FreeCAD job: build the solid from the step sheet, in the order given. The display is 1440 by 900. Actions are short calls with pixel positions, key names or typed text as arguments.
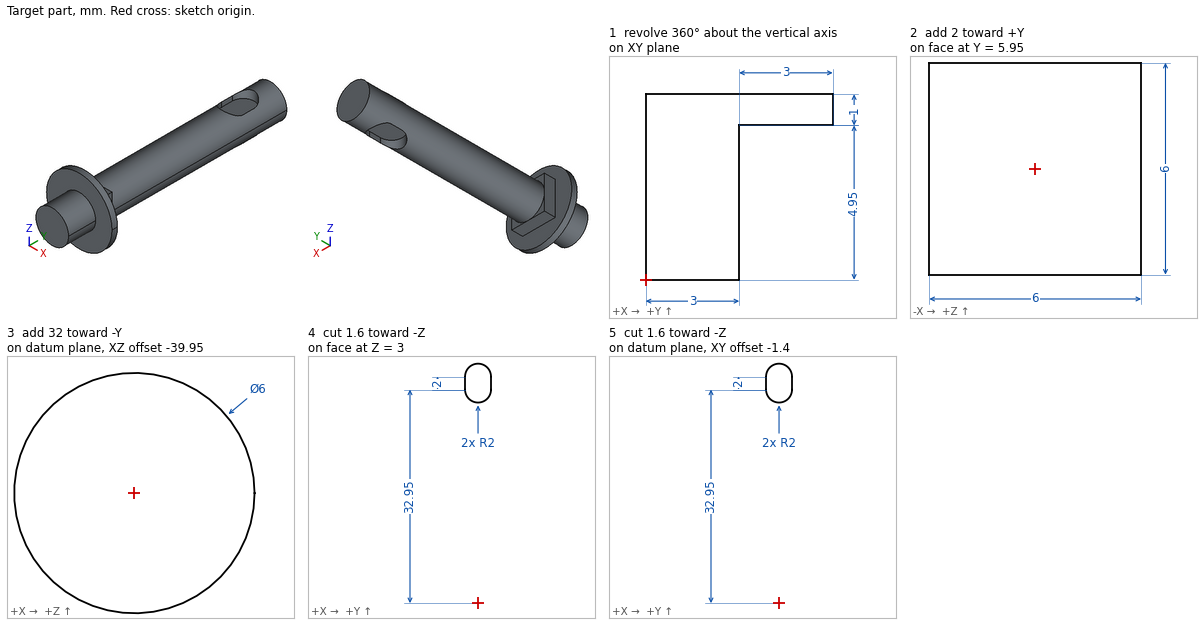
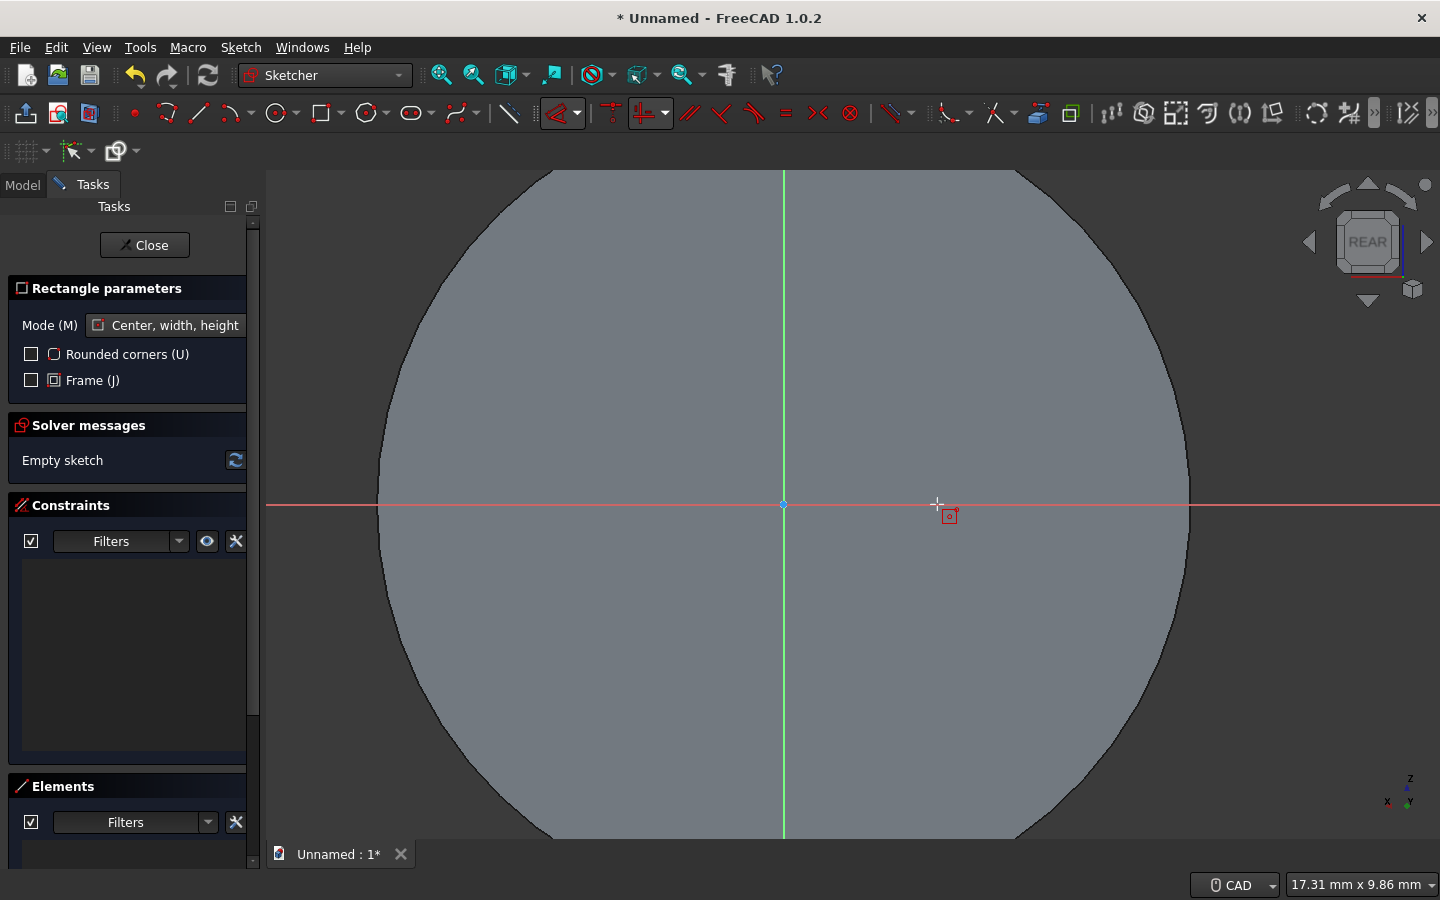
click(784, 504)
click(987, 301)
key(Escape)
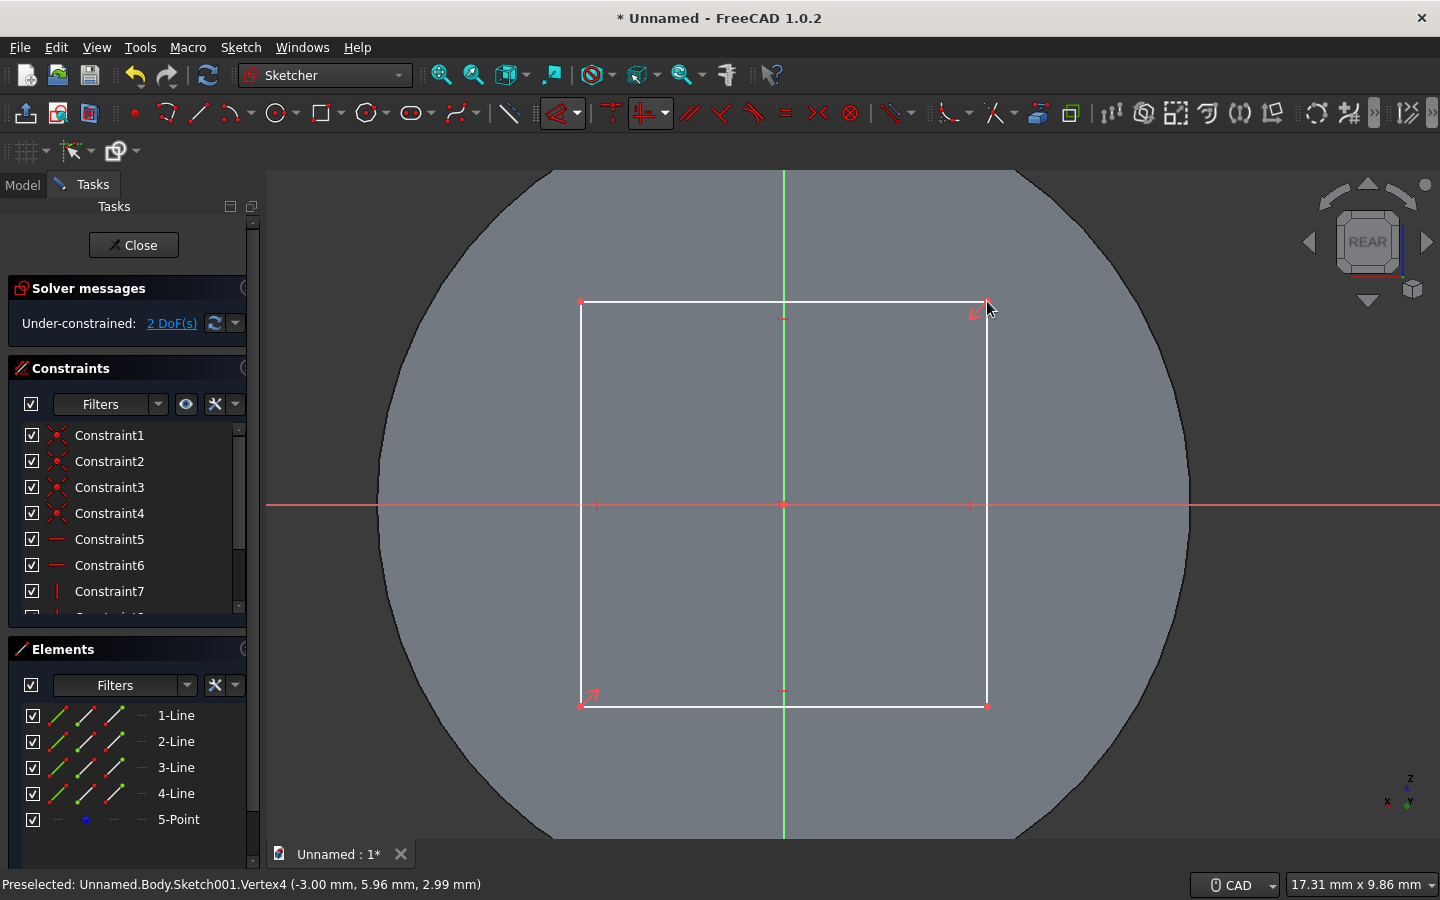
click(703, 707)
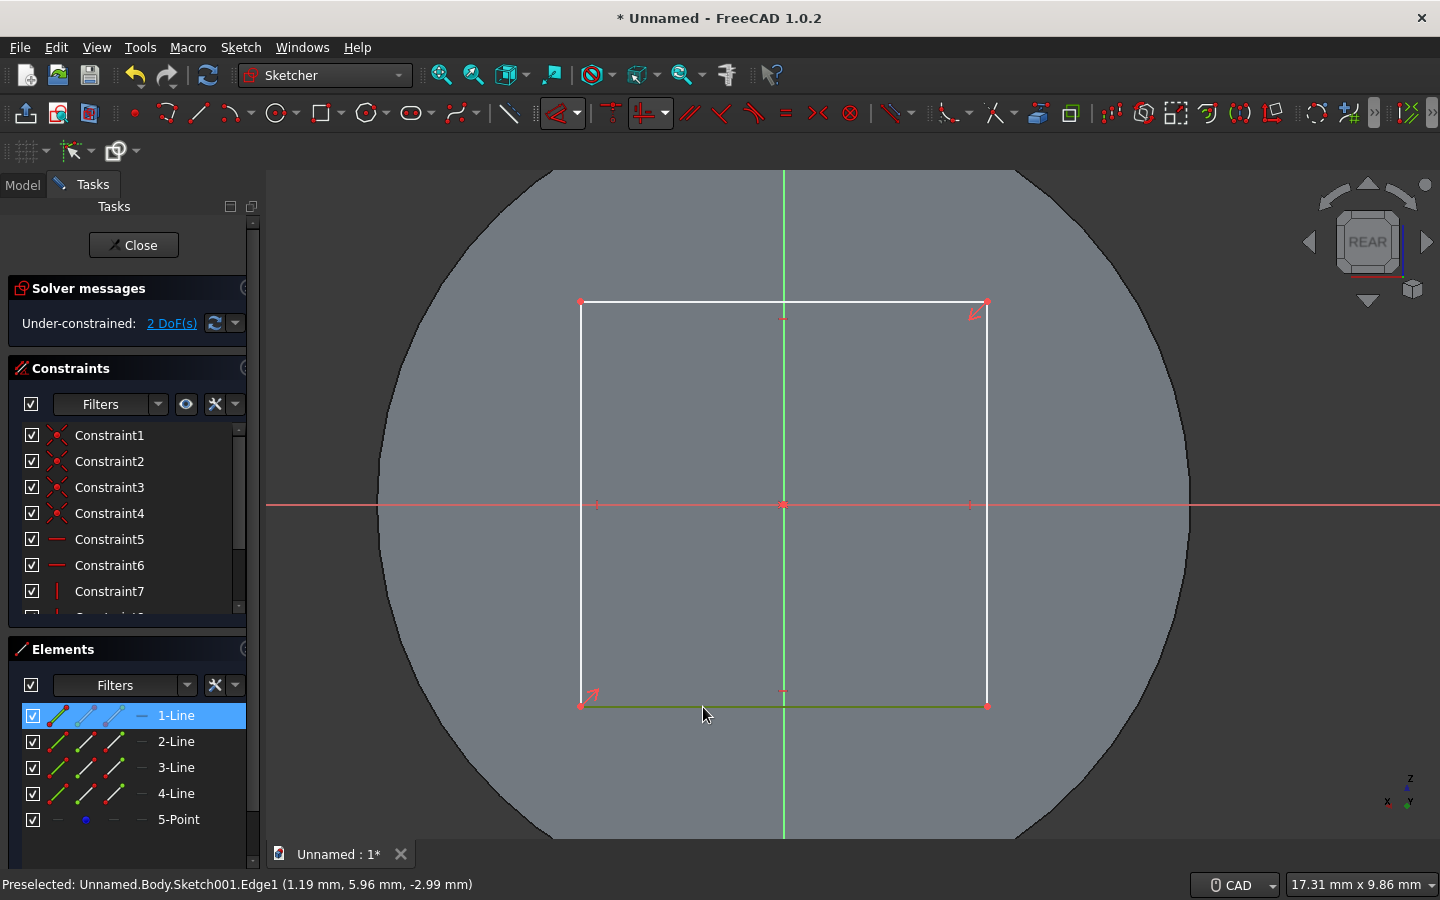
click(580, 114)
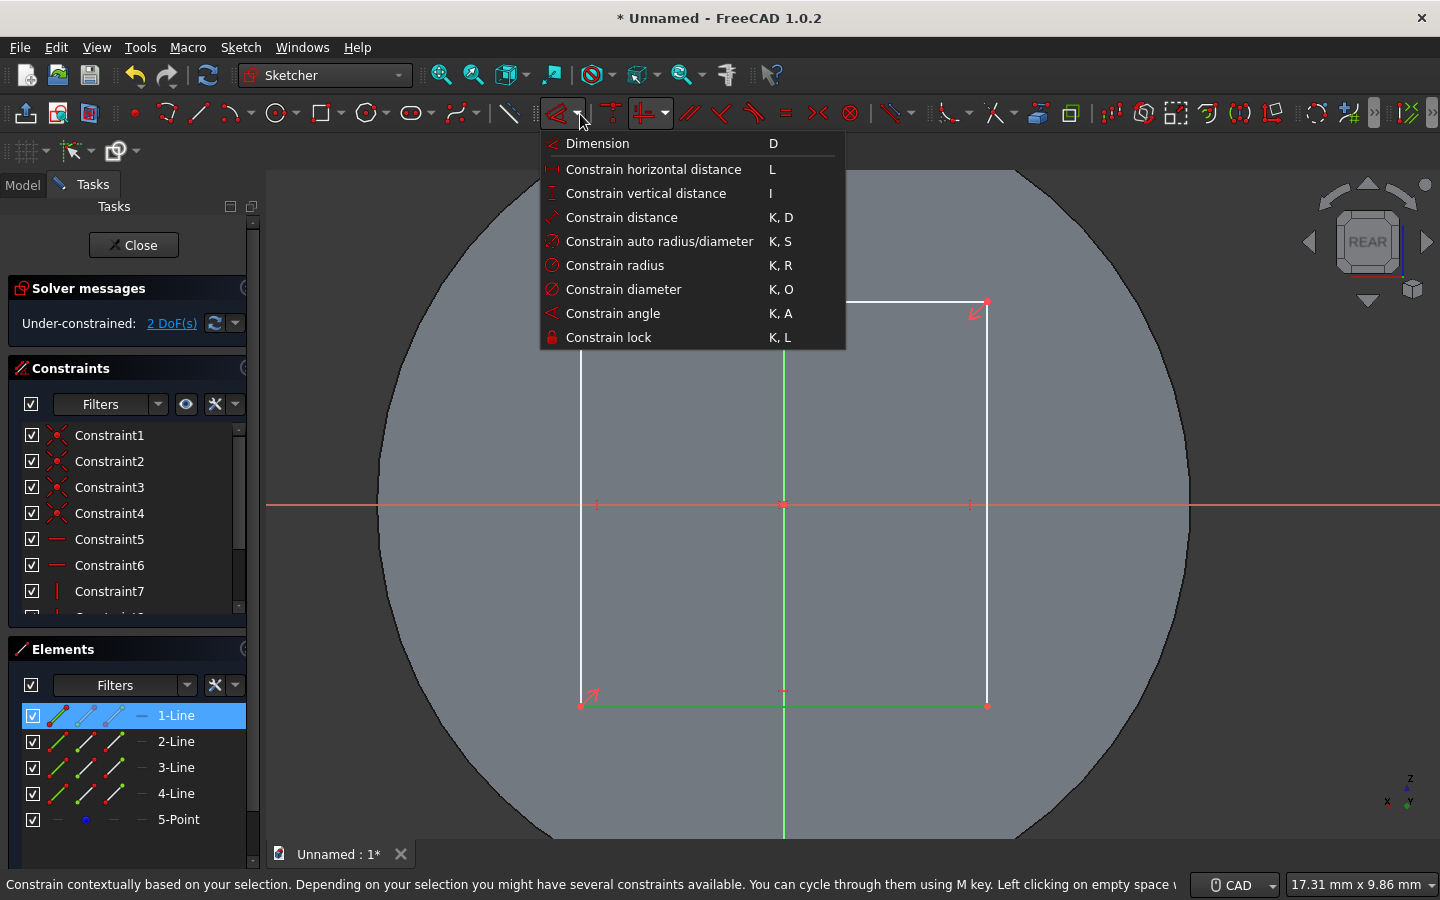
click(693, 169)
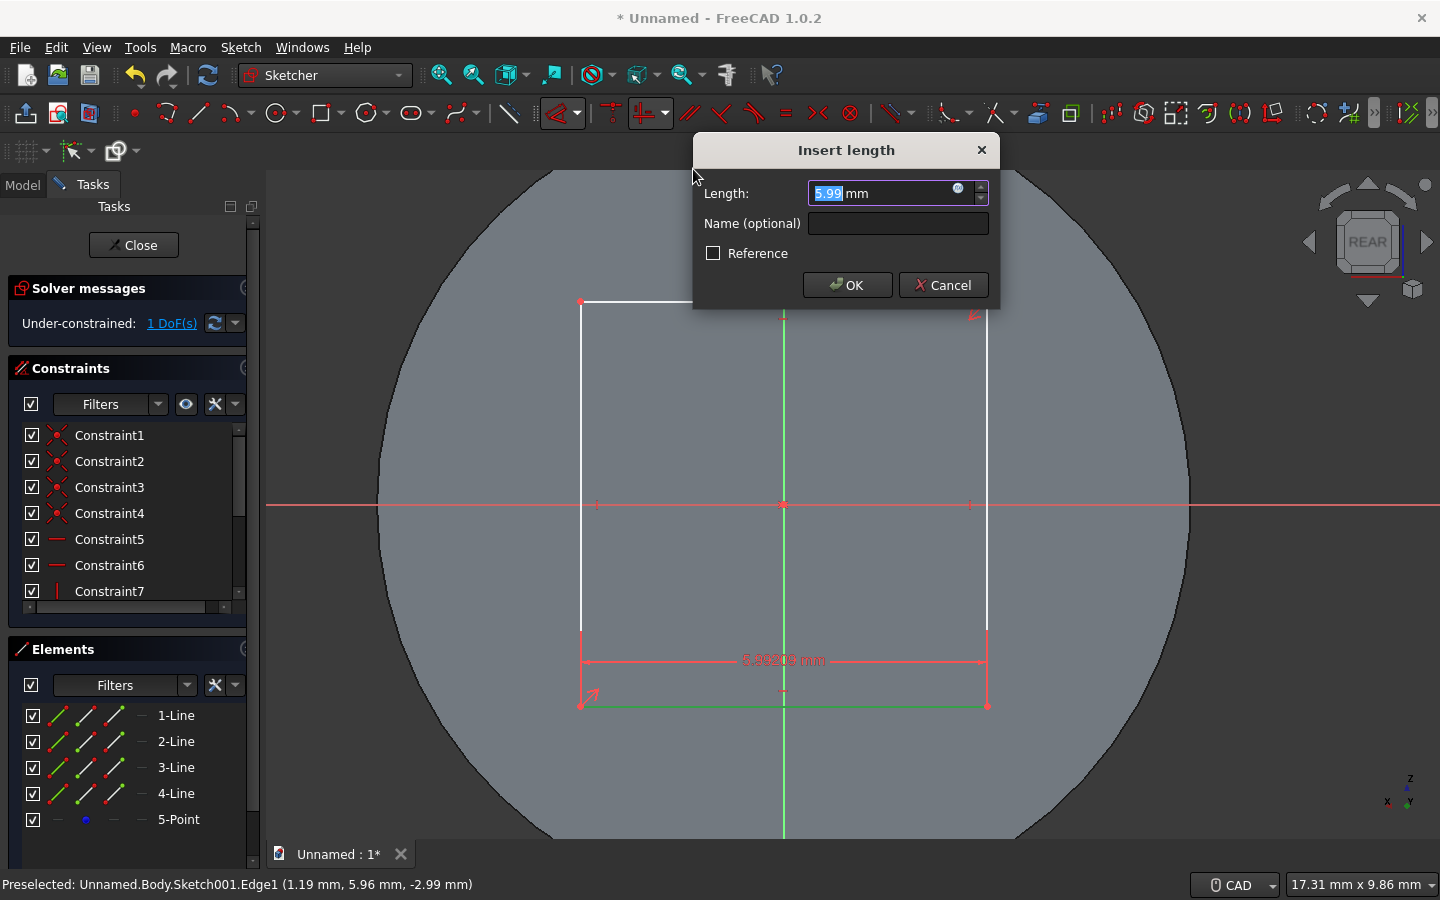
text(6)
key(Return)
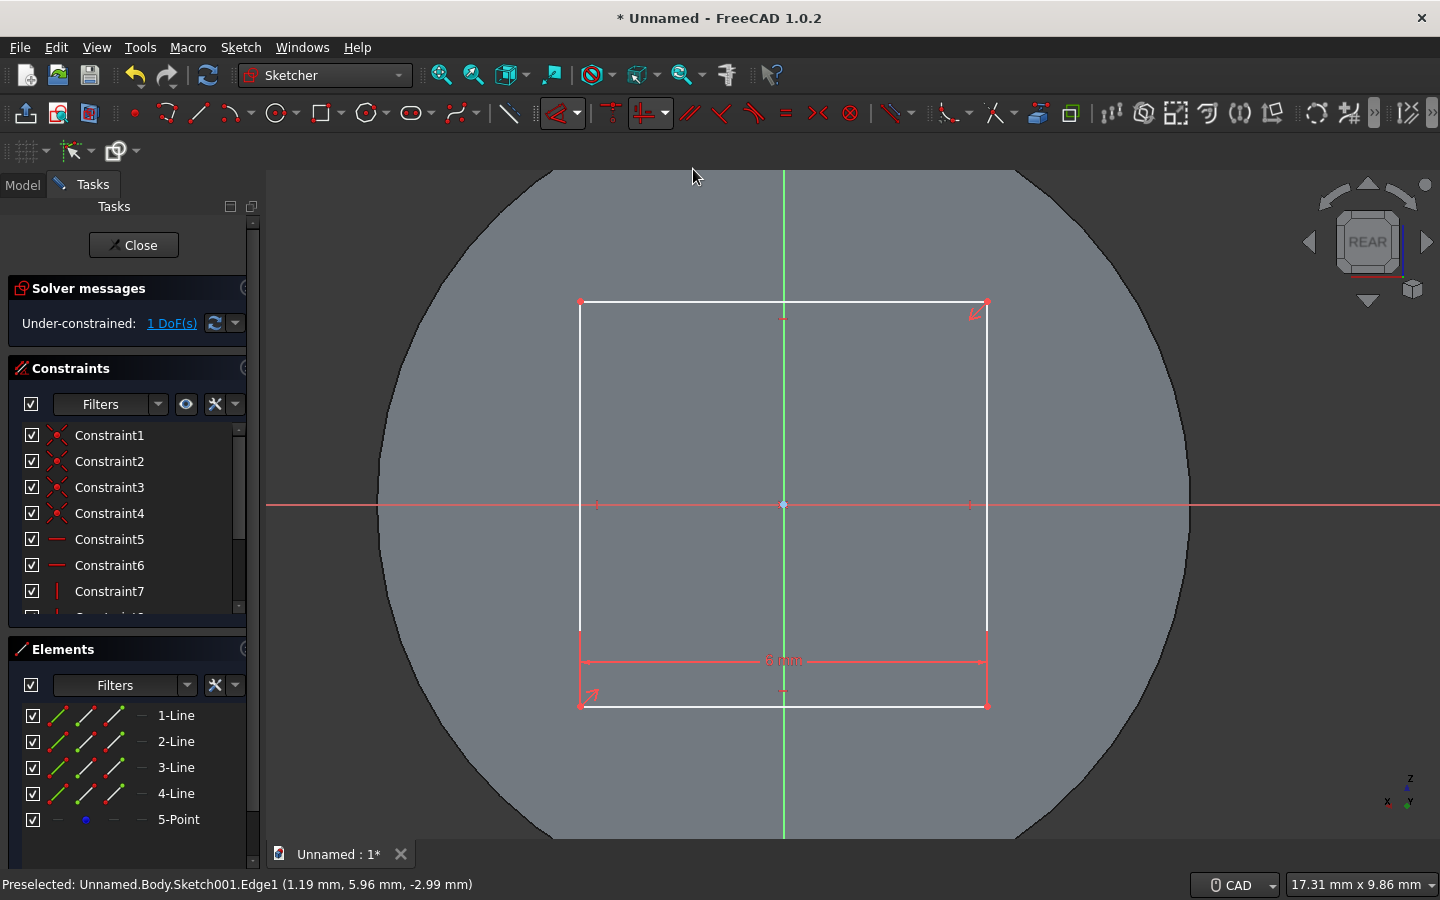
click(987, 585)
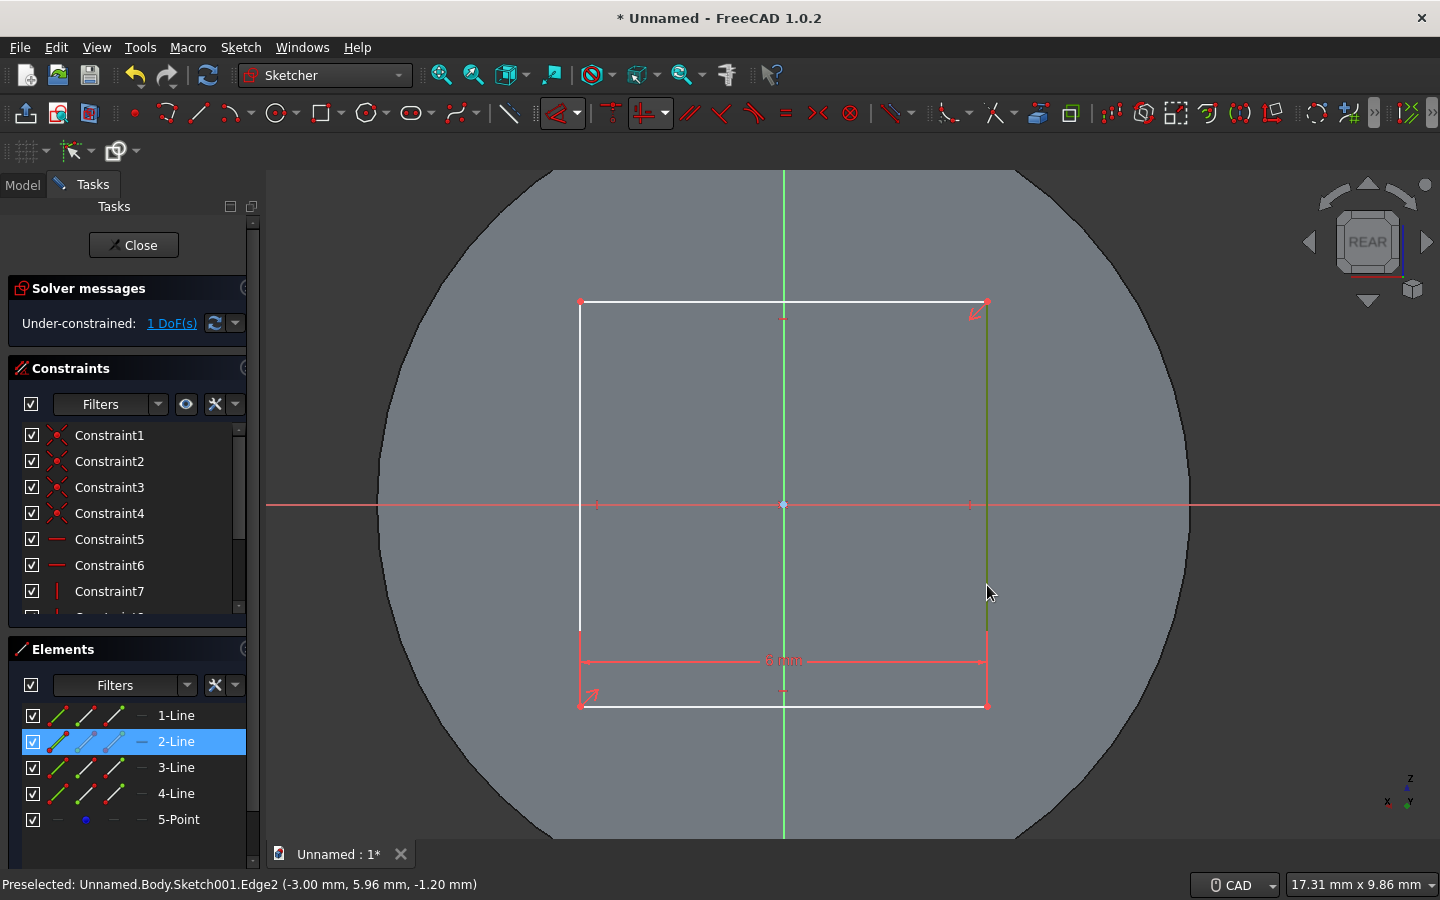
click(580, 114)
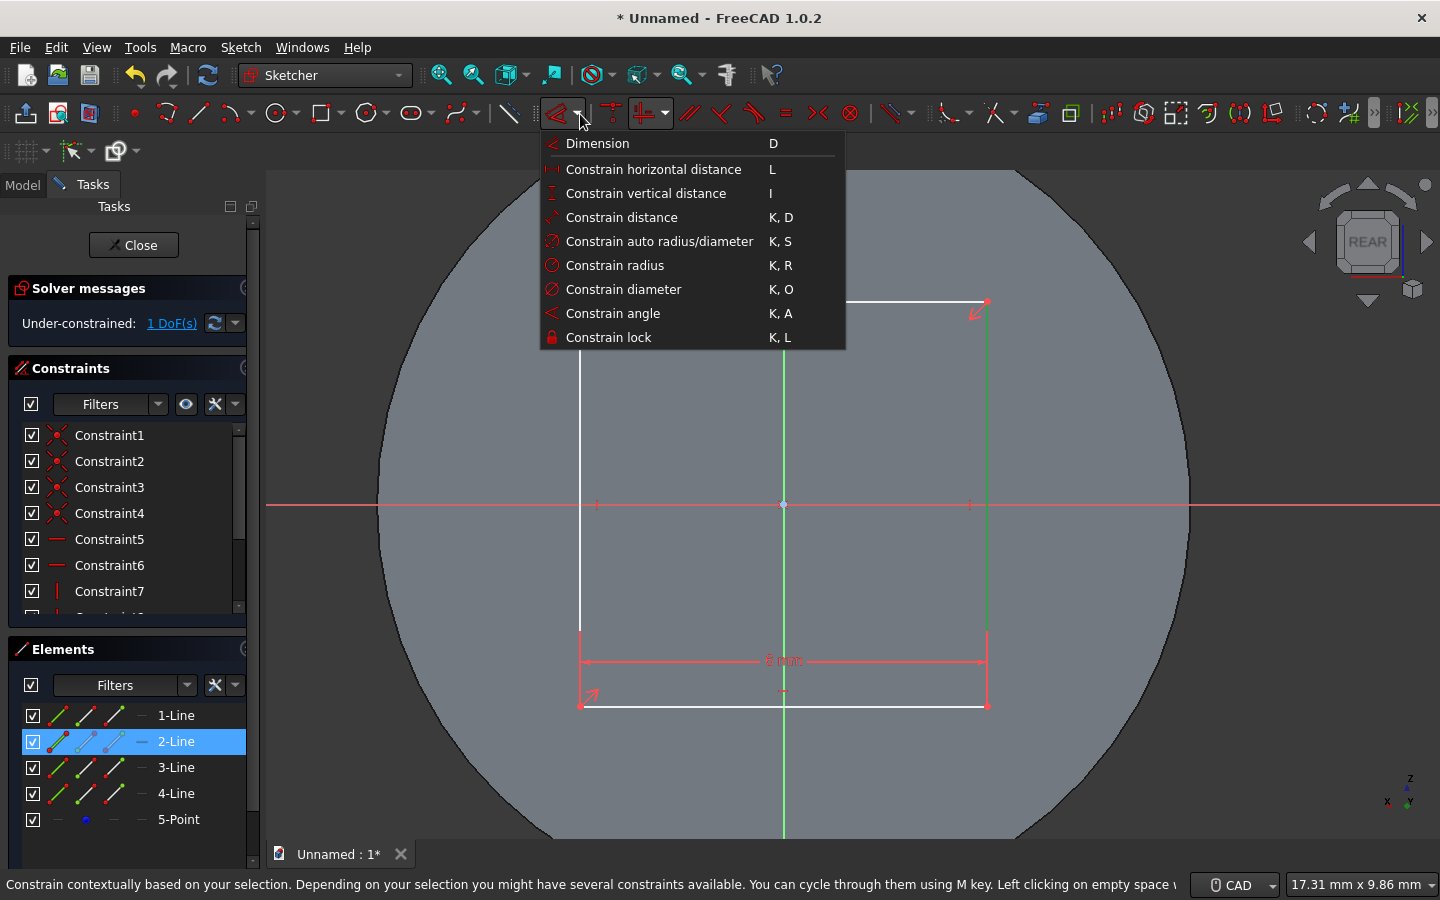
click(693, 193)